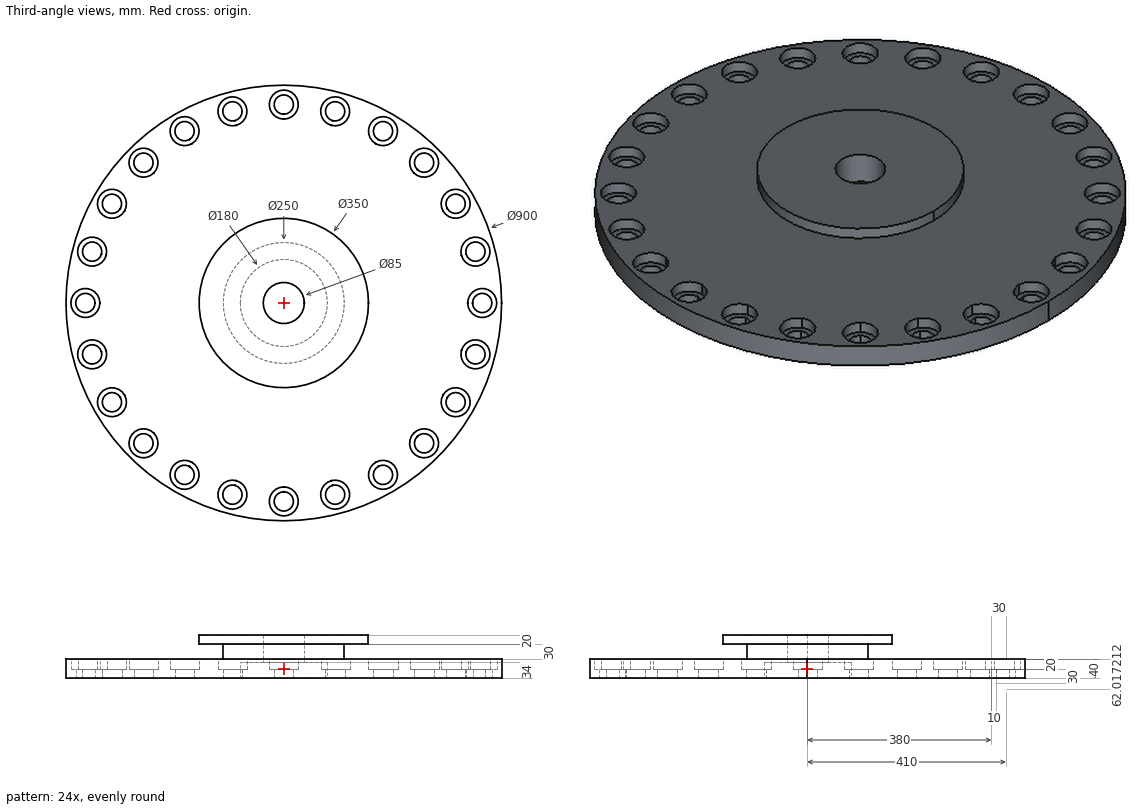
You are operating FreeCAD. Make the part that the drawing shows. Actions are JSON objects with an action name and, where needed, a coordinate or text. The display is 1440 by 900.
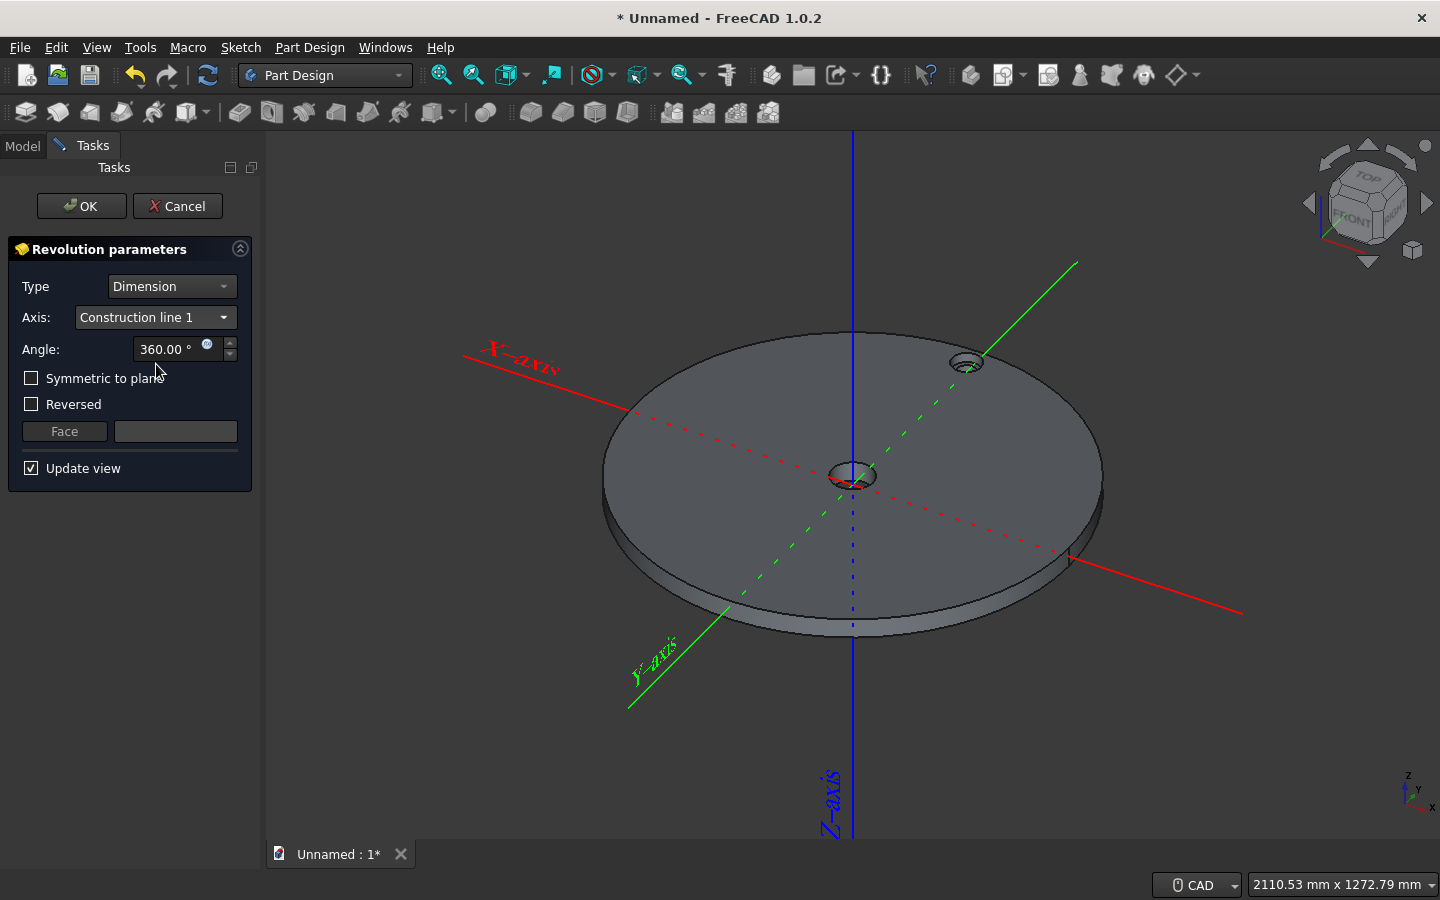
{"action": "left_click", "coordinate": [82, 206]}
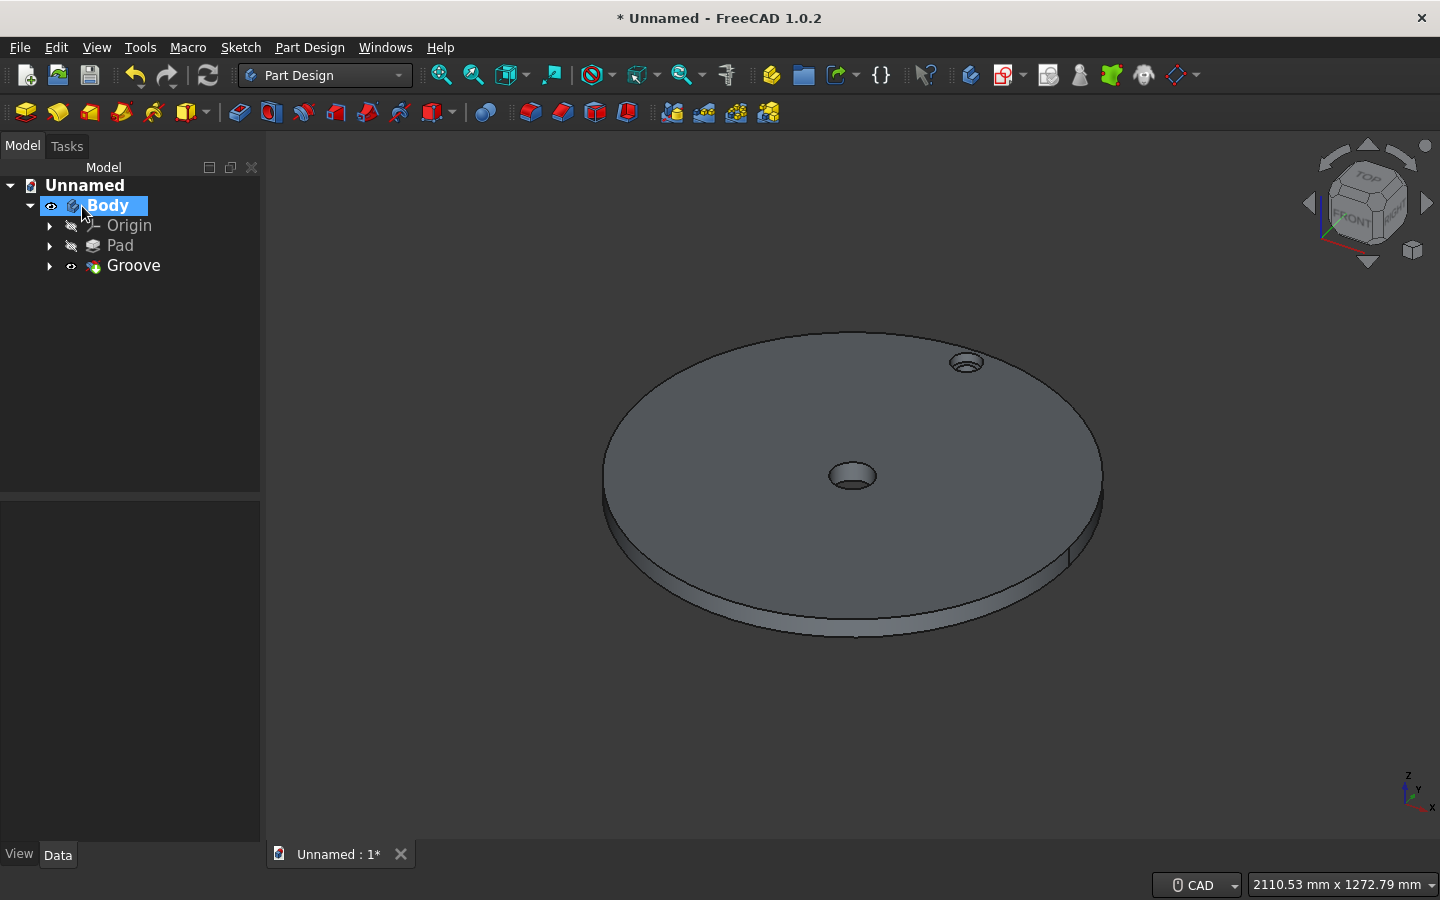
{"action": "left_click", "coordinate": [116, 266]}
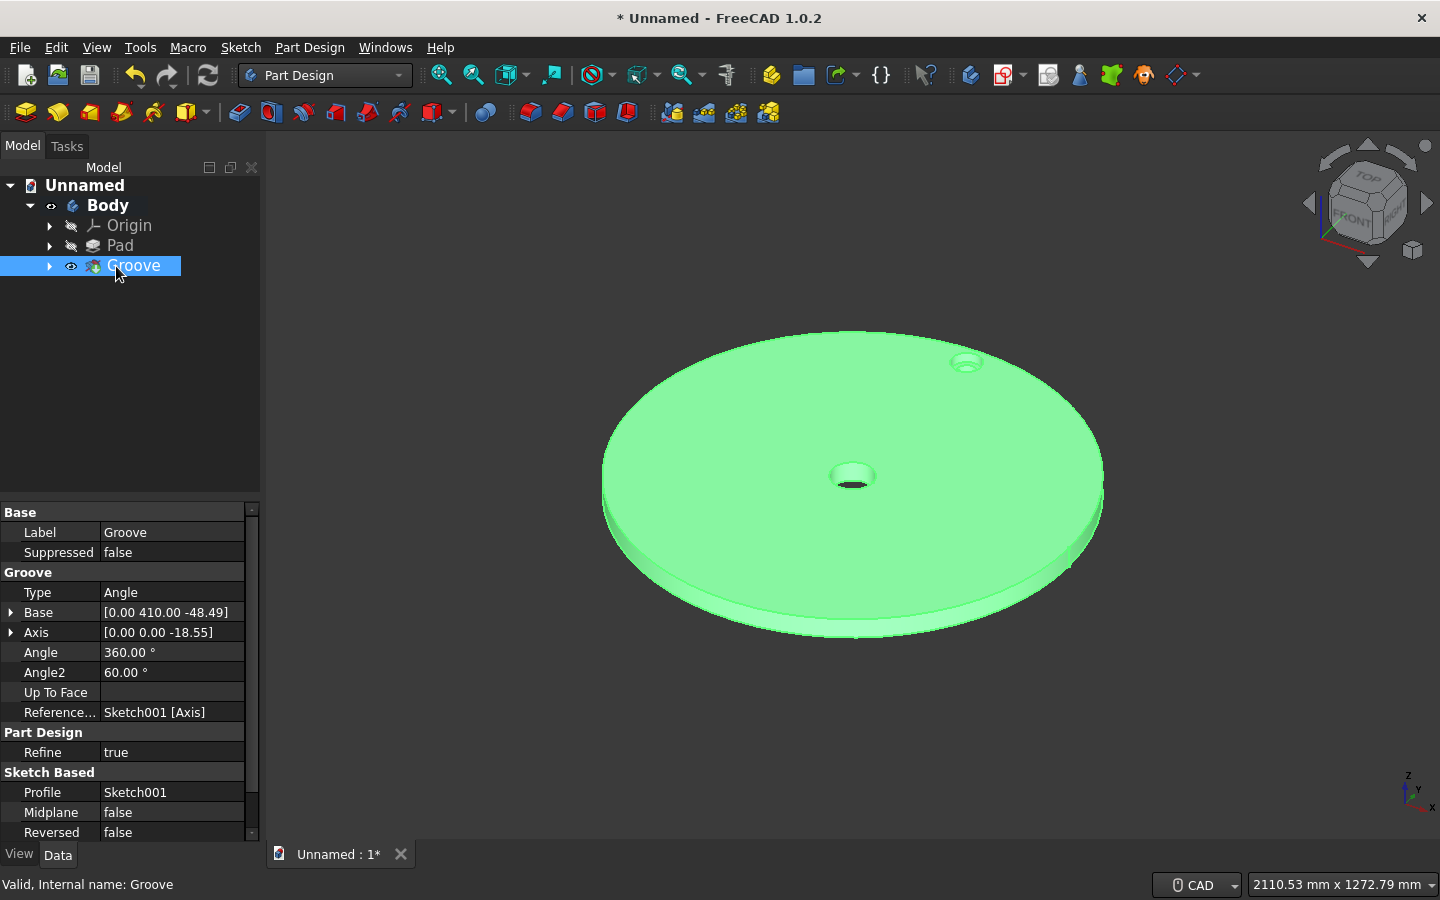
{"action": "left_click", "coordinate": [736, 112]}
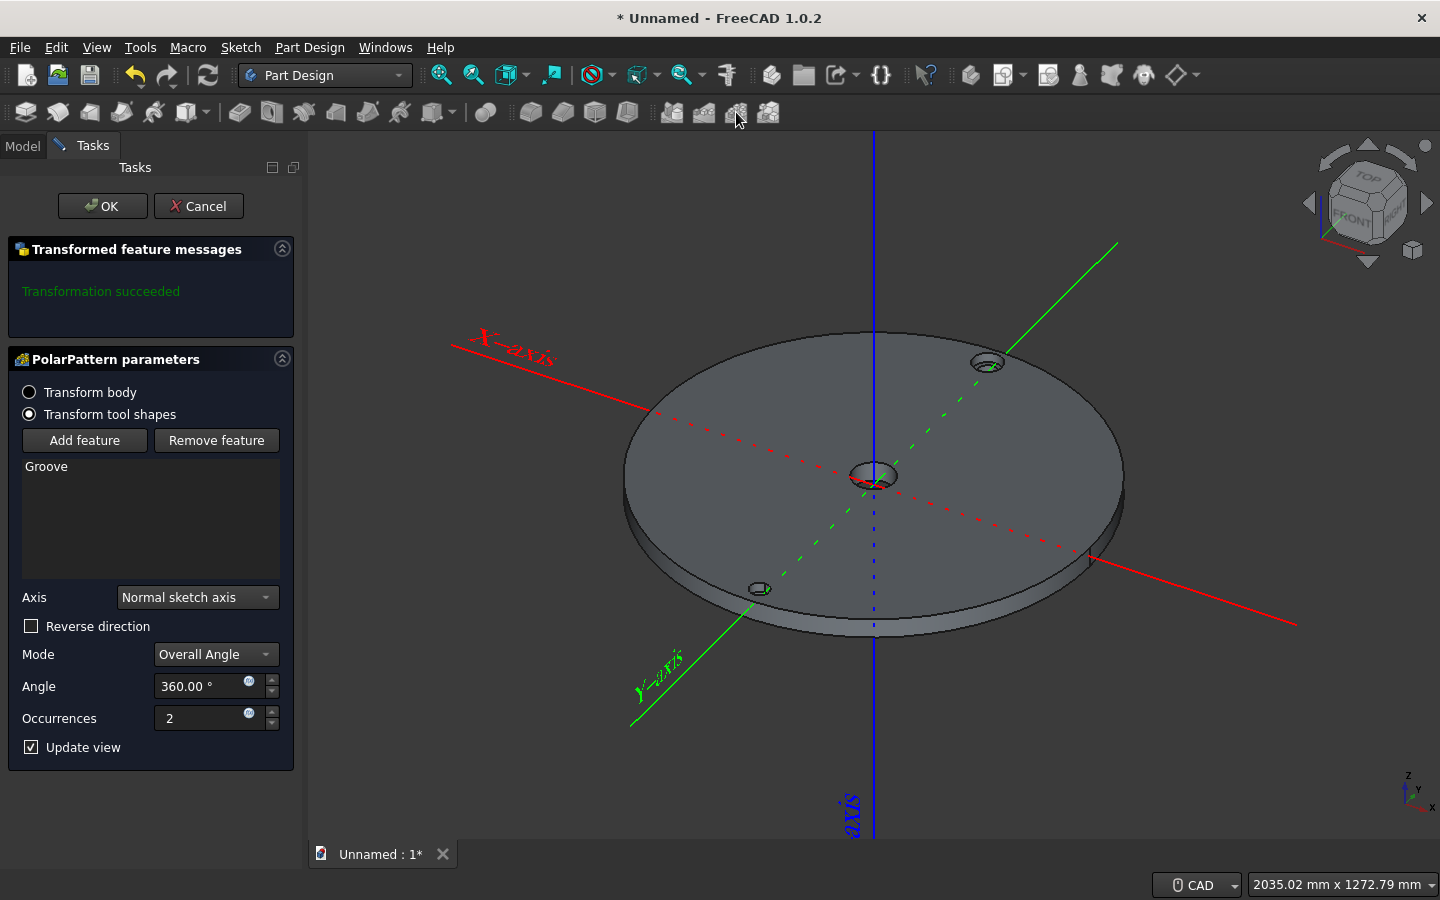
{"action": "left_click", "coordinate": [198, 598]}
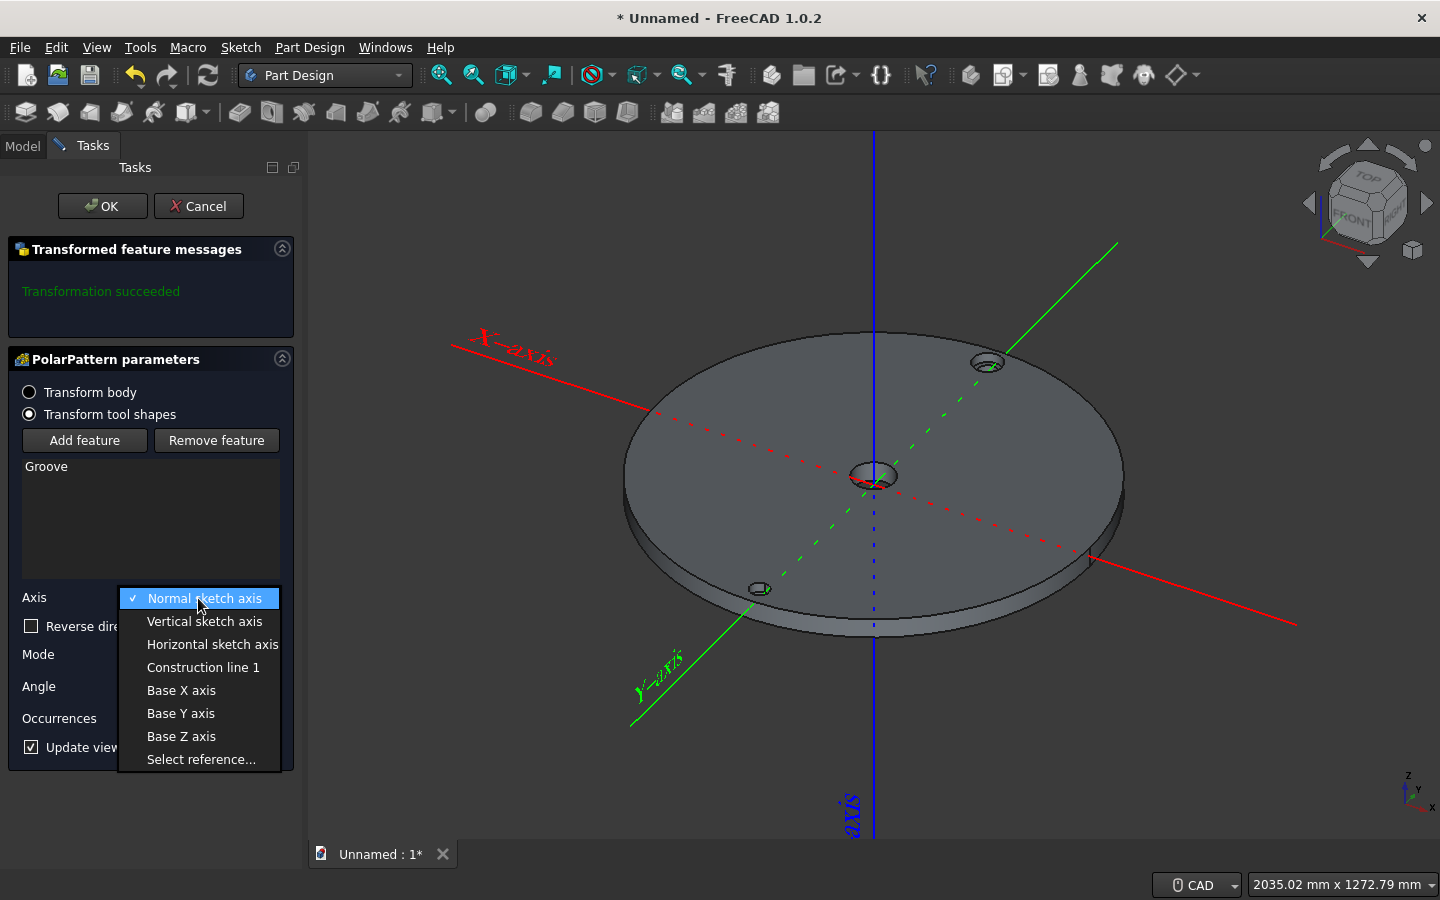
{"action": "left_click", "coordinate": [198, 736]}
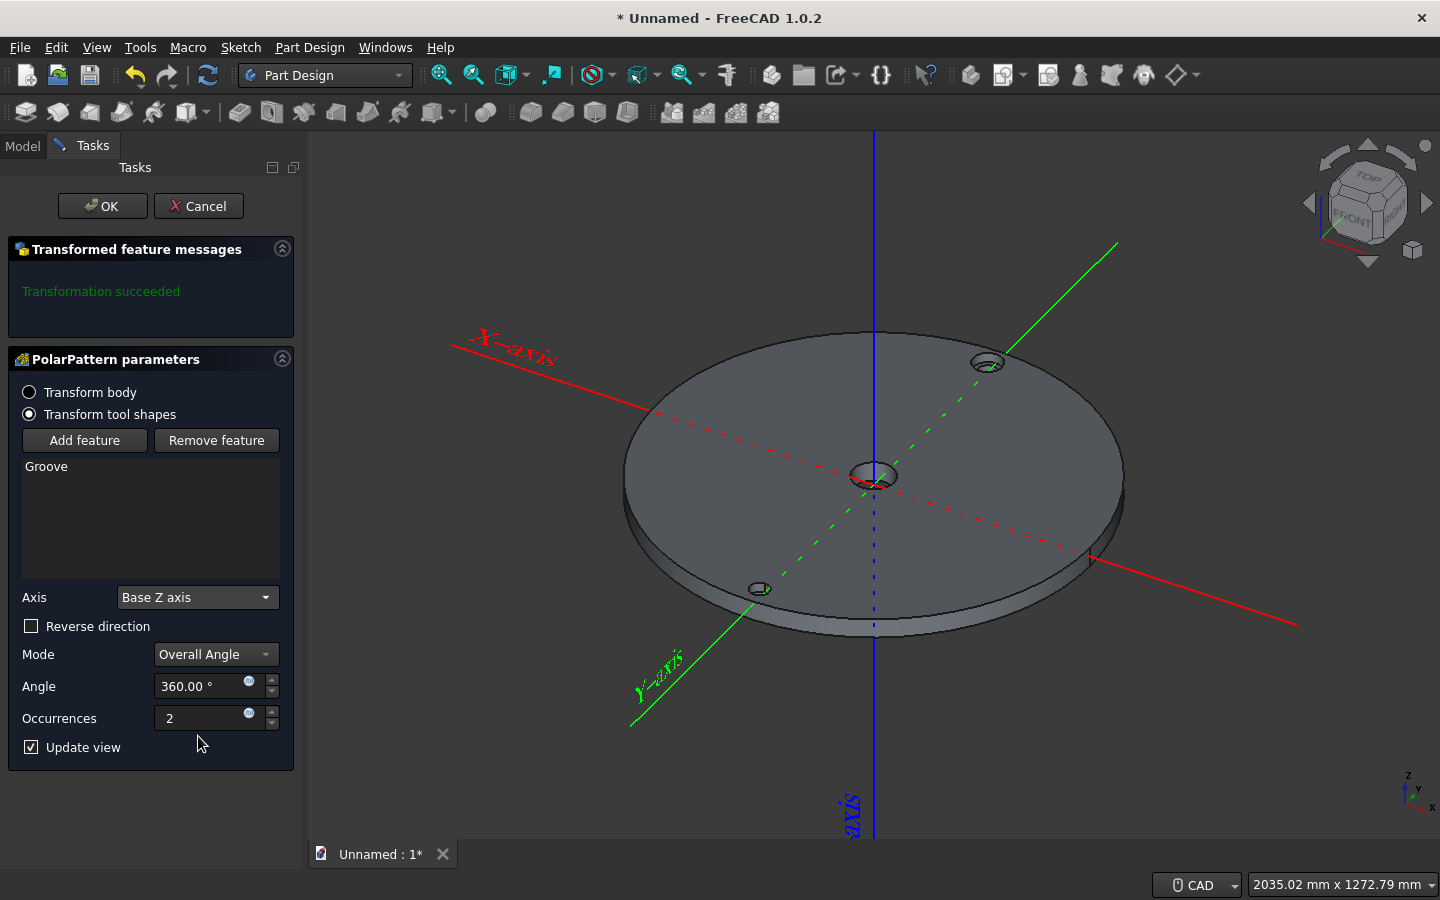
{"action": "triple_click", "coordinate": [209, 718]}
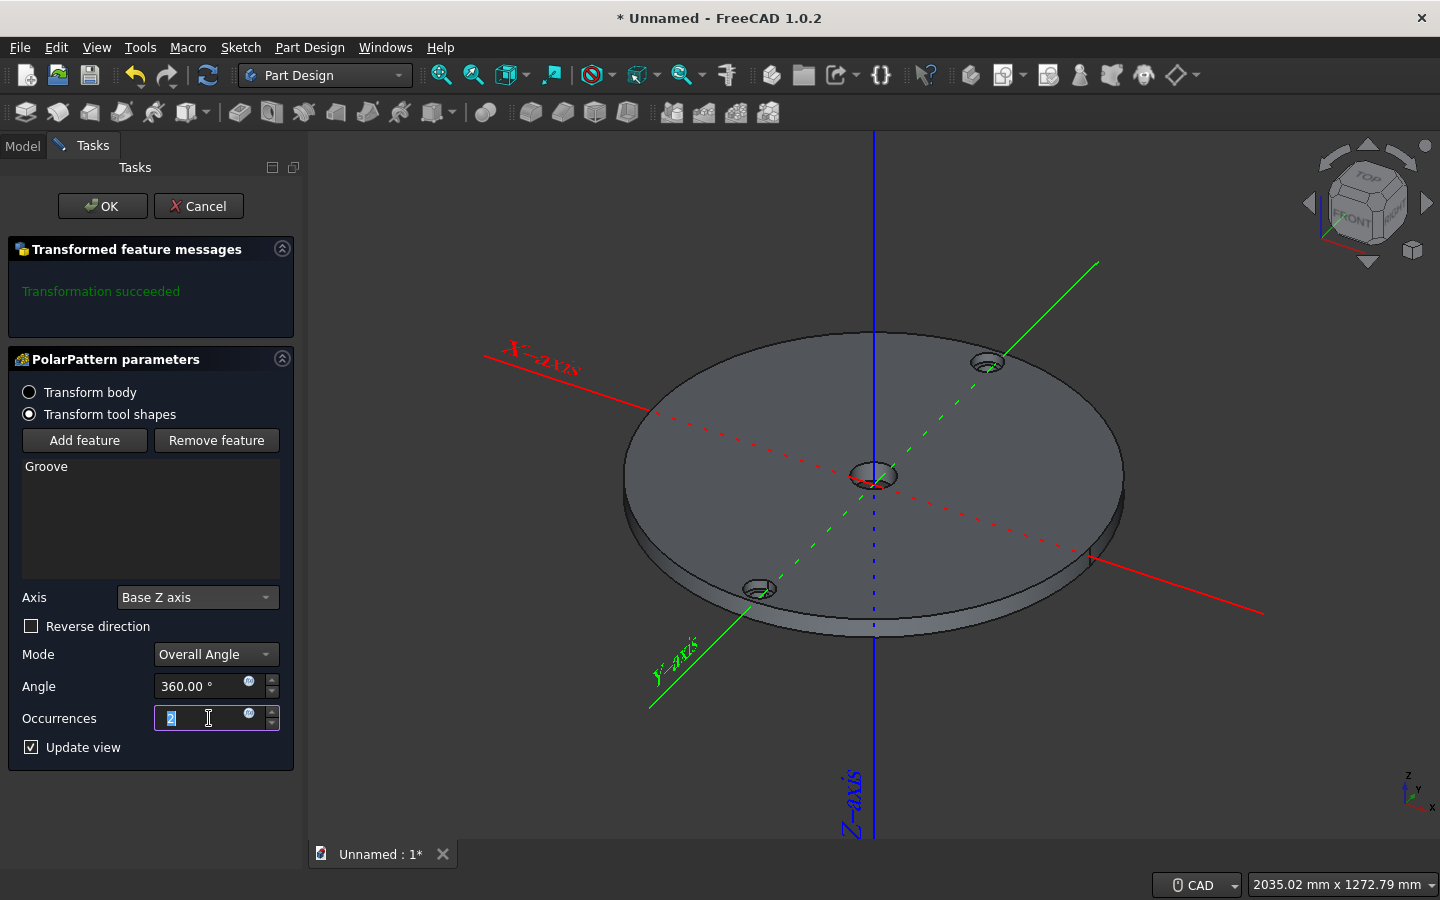
{"action": "type", "text": "24"}
{"action": "key", "text": "Tab"}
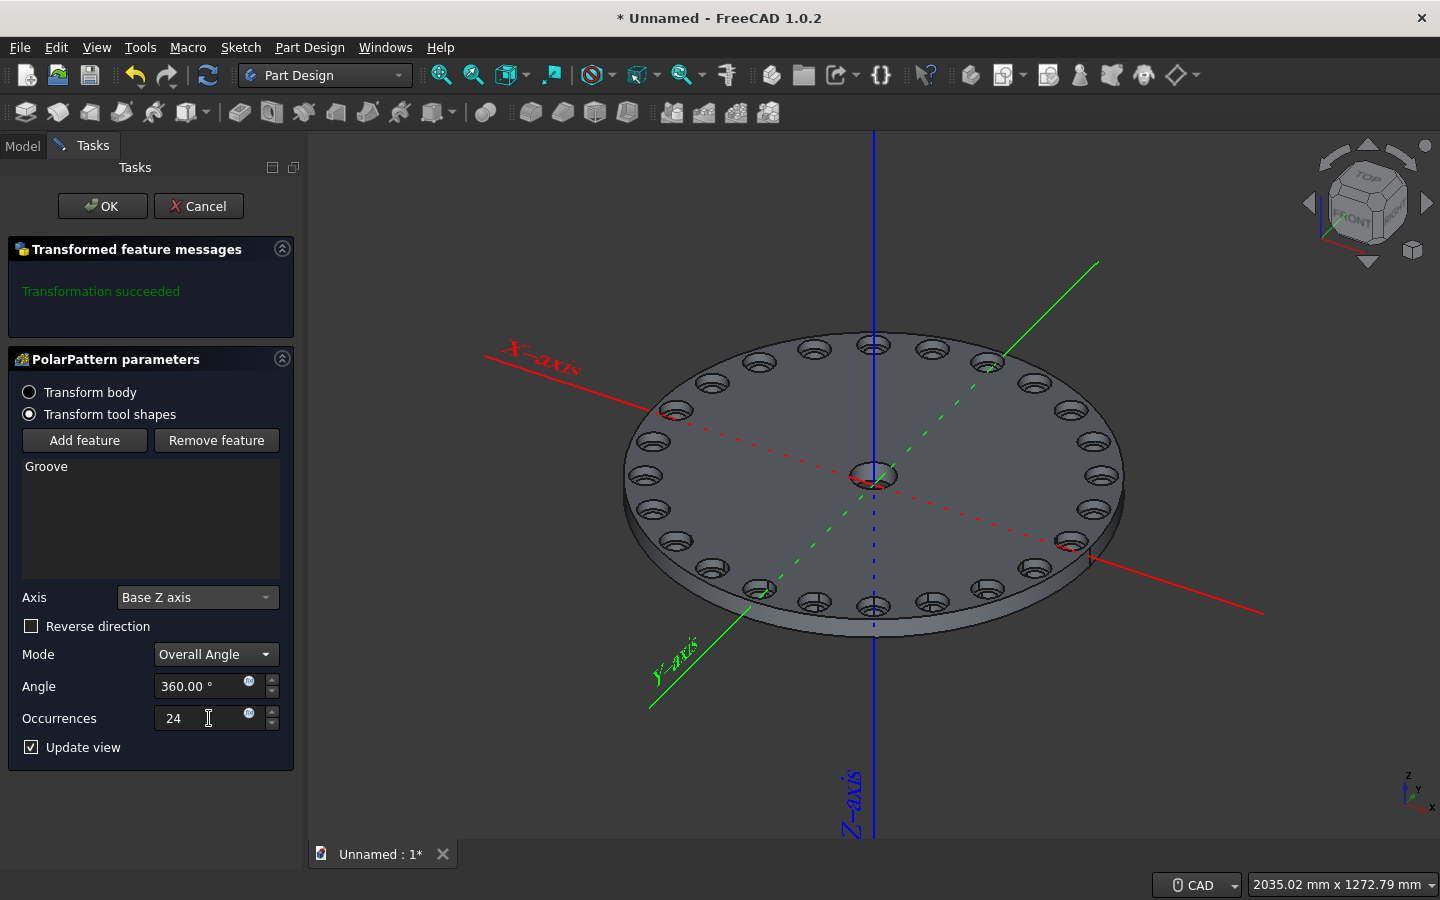
{"action": "left_click", "coordinate": [103, 206]}